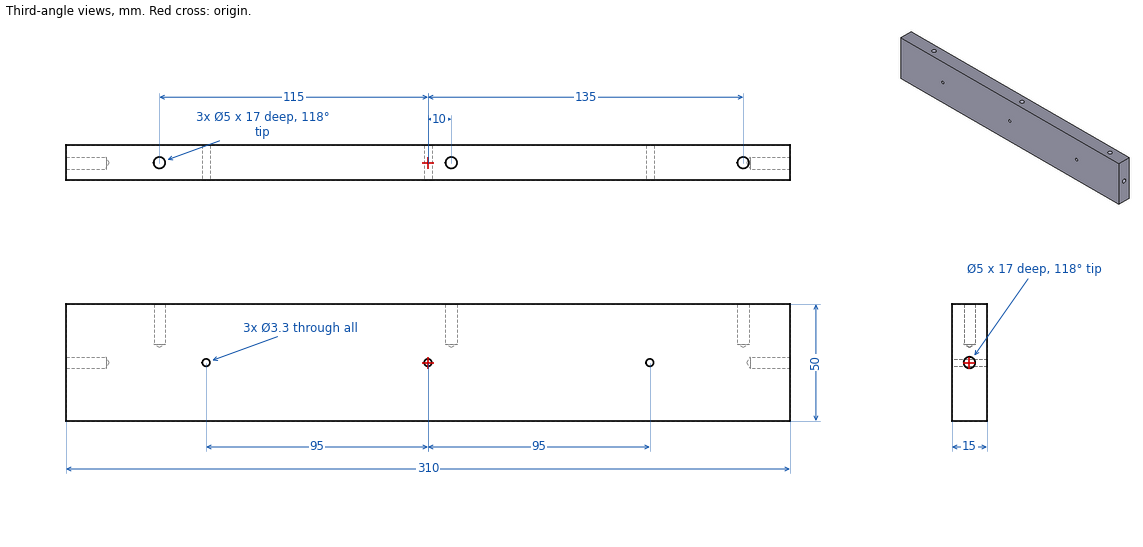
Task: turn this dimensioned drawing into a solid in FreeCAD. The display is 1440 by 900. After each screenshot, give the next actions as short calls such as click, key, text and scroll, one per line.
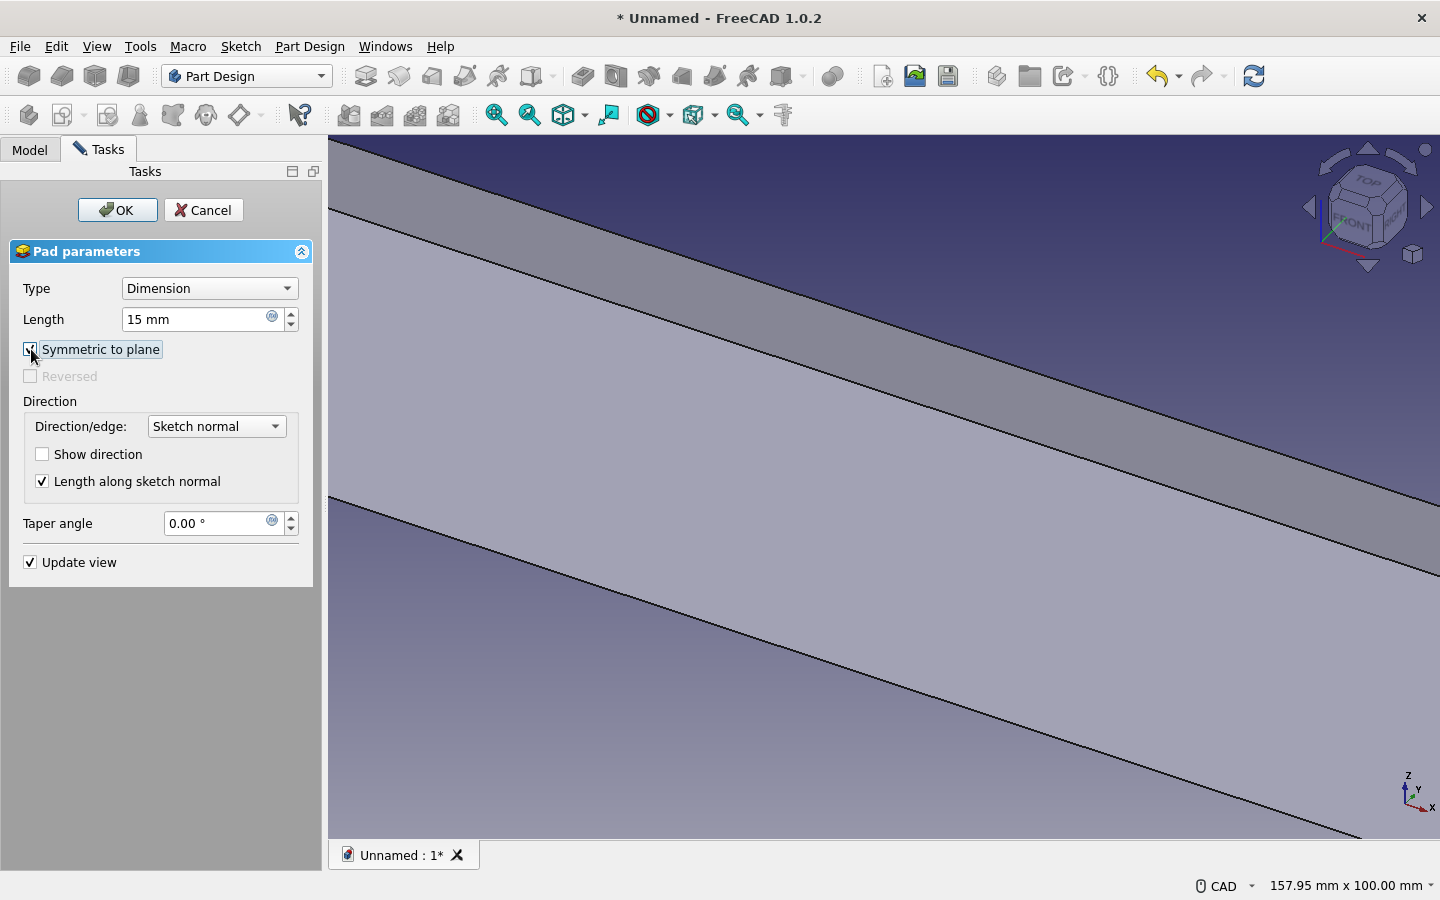
click(118, 210)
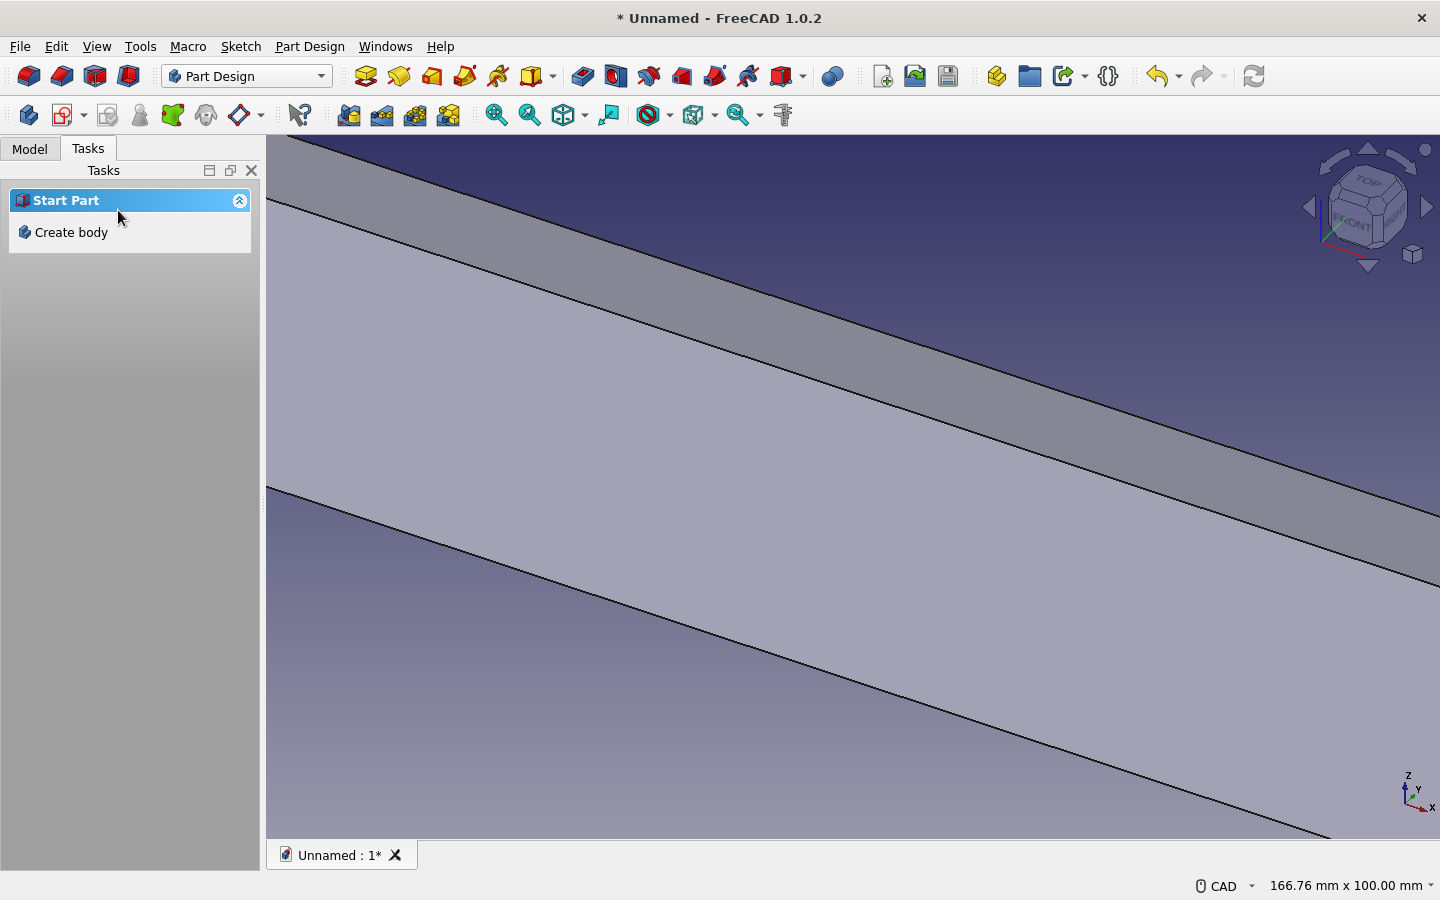
click(497, 116)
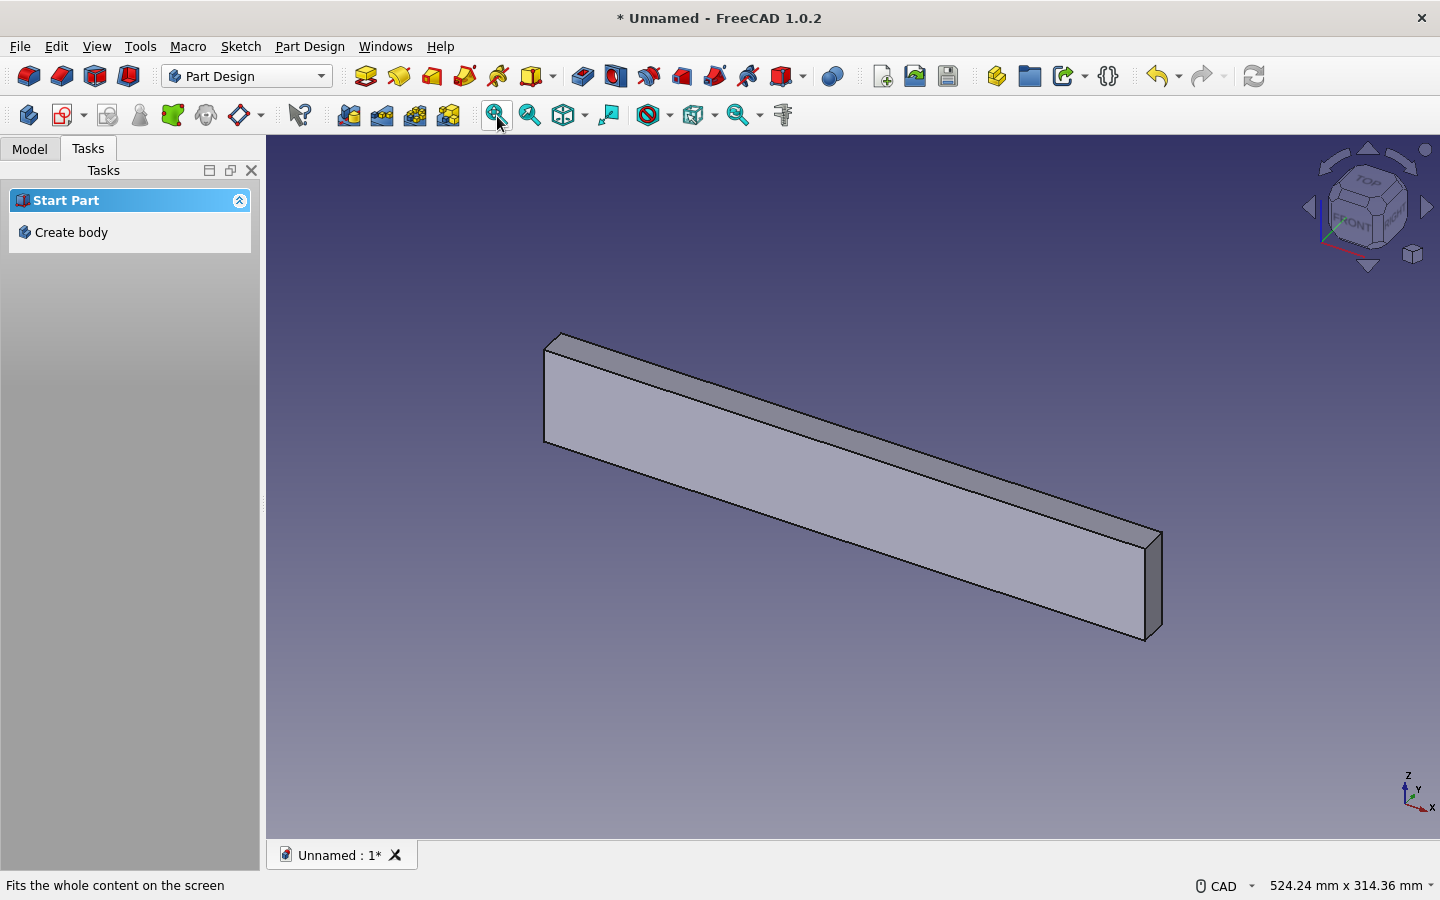
click(1111, 525)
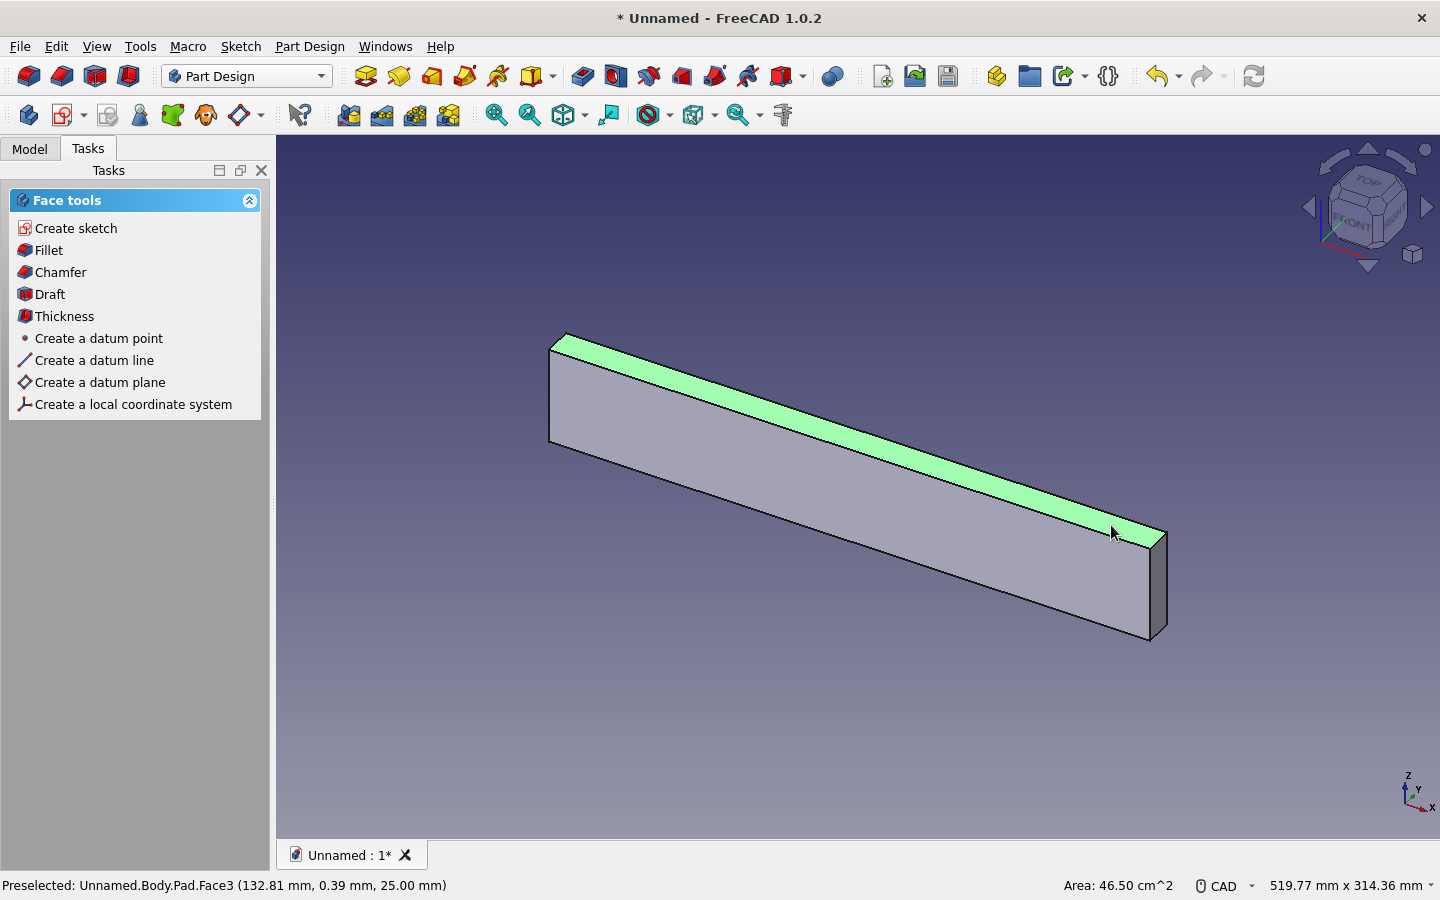
click(62, 116)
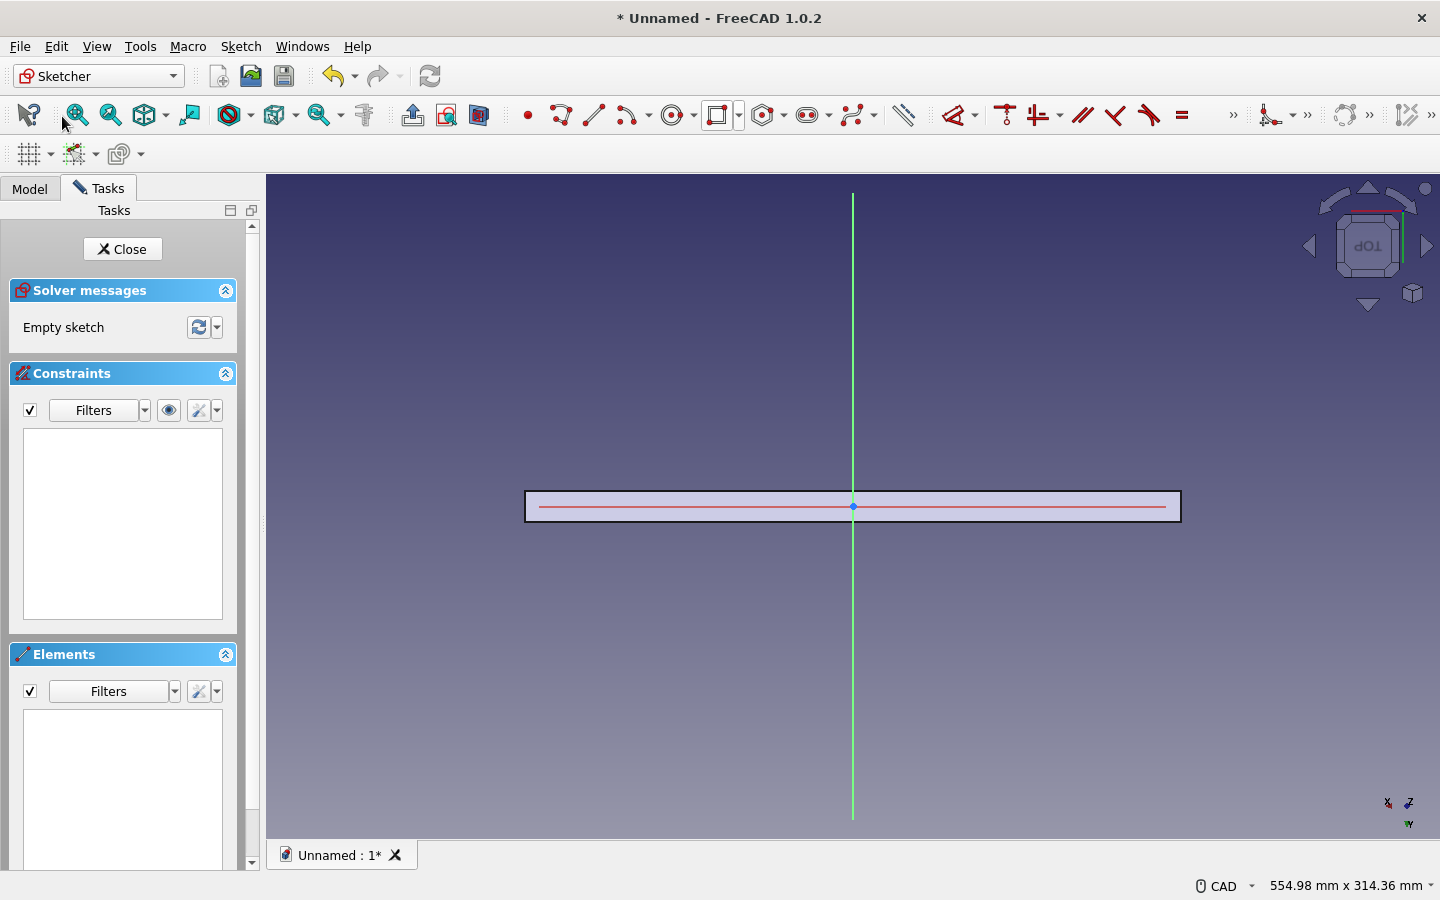
click(672, 116)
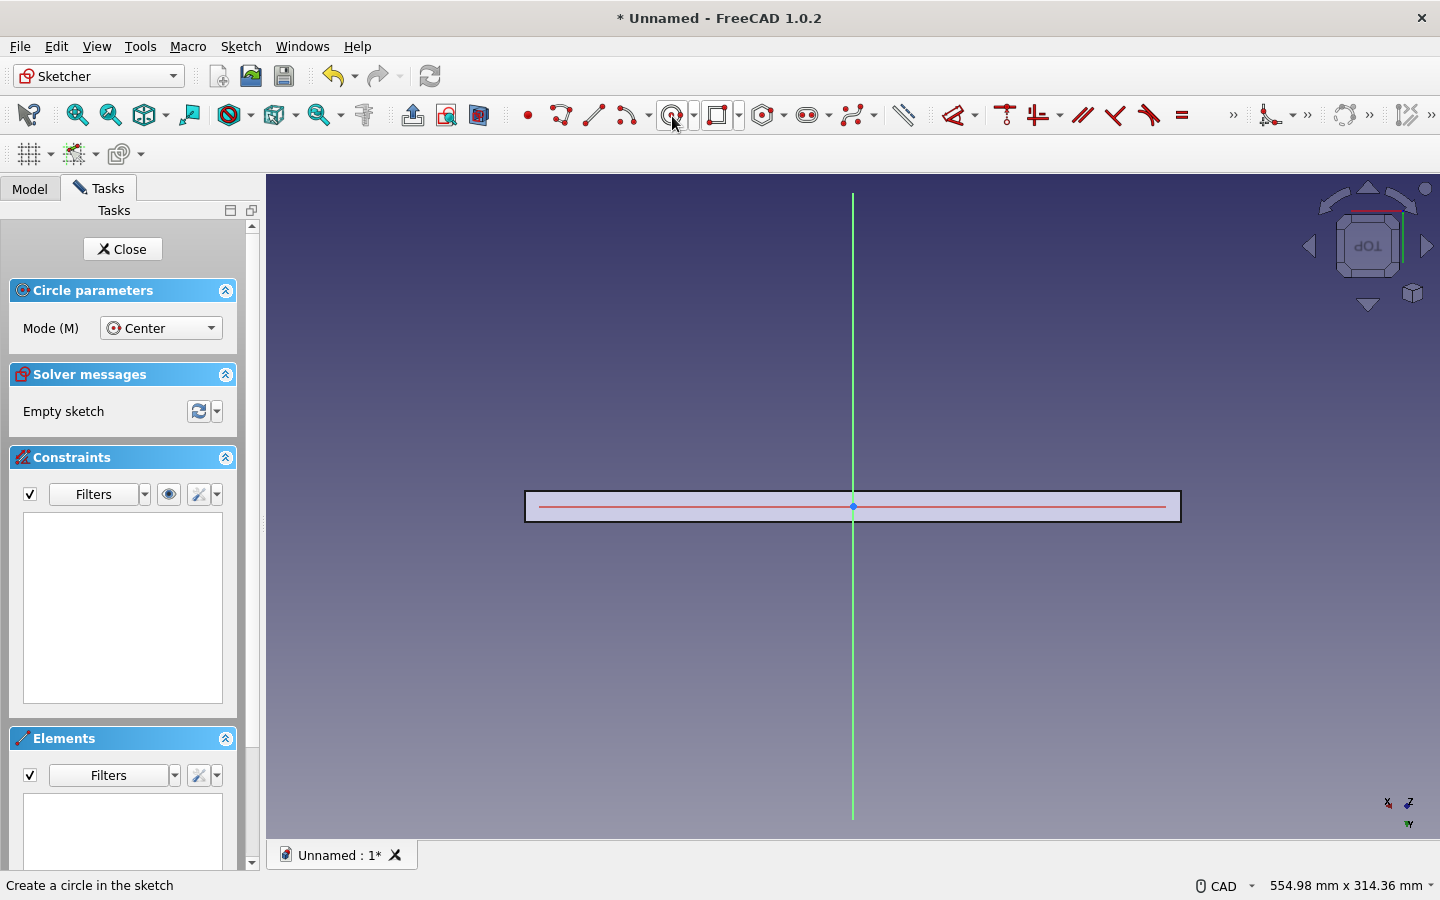
scroll(1096, 506, up, 8)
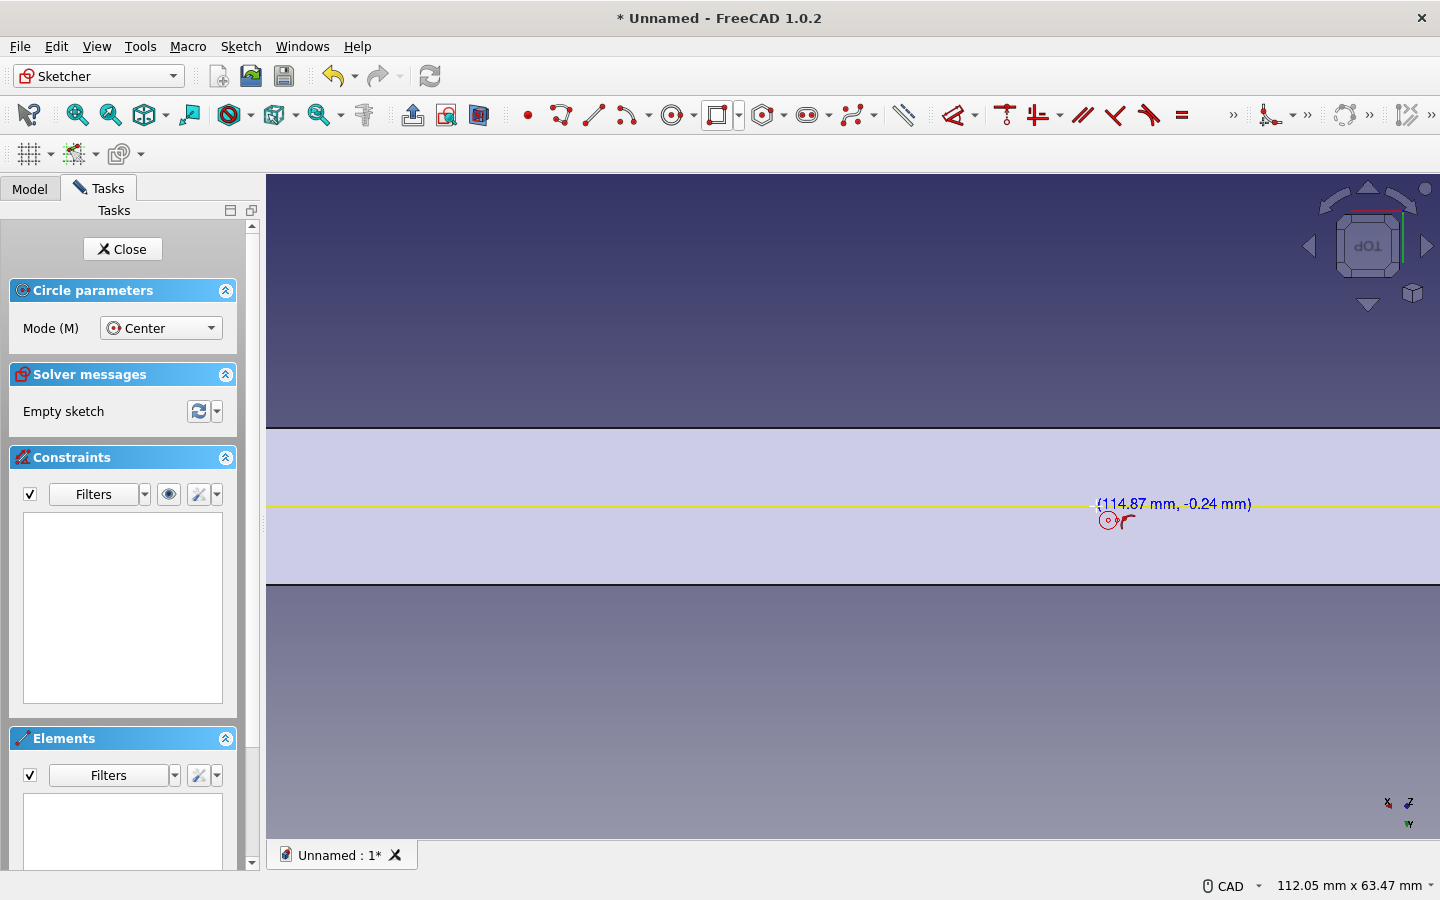
scroll(1112, 506, down, 7)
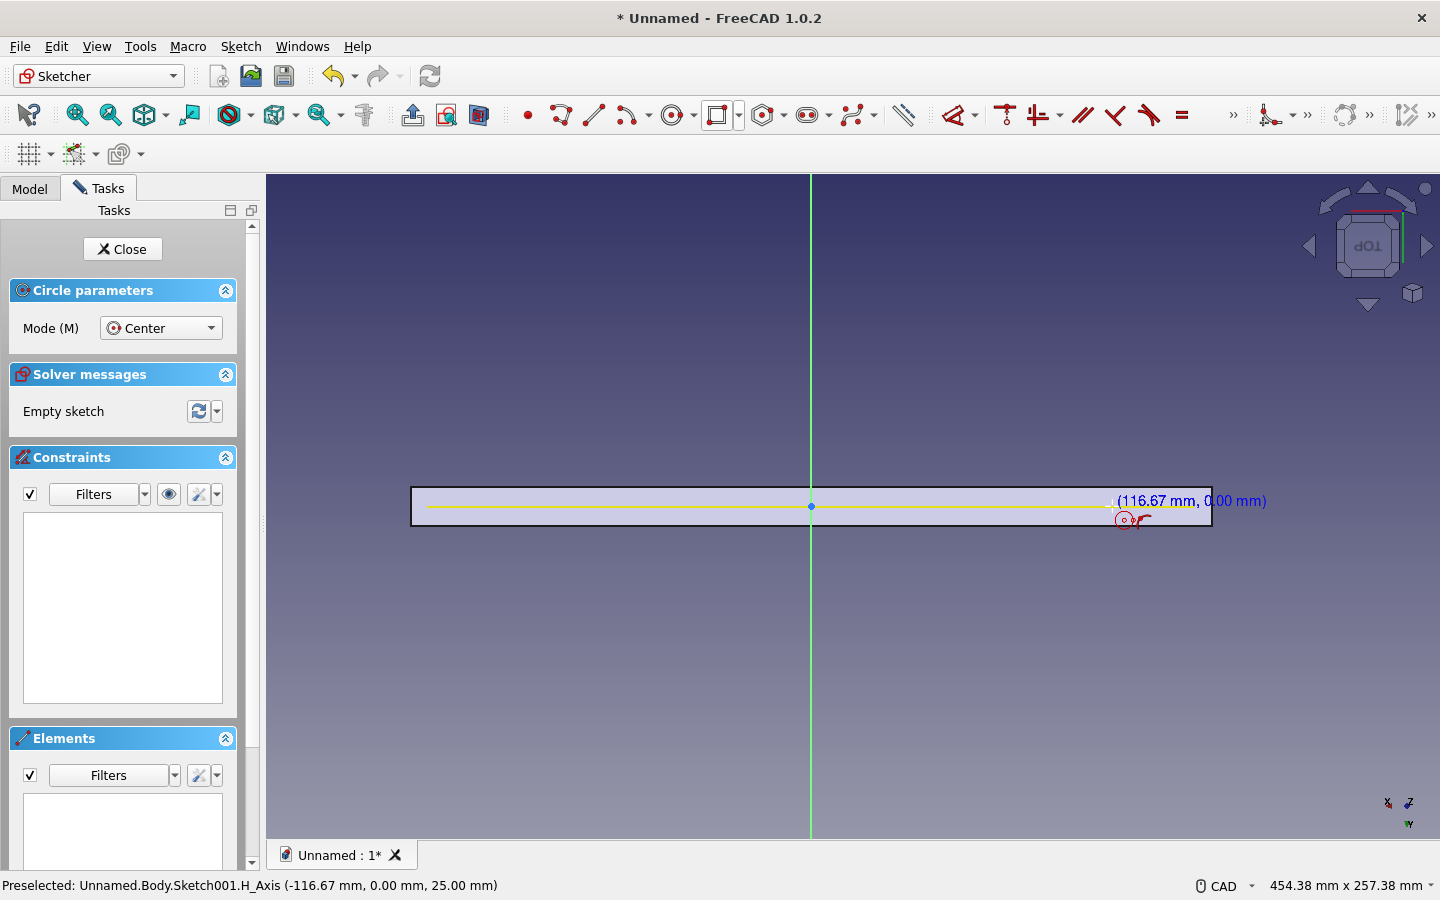
click(1108, 506)